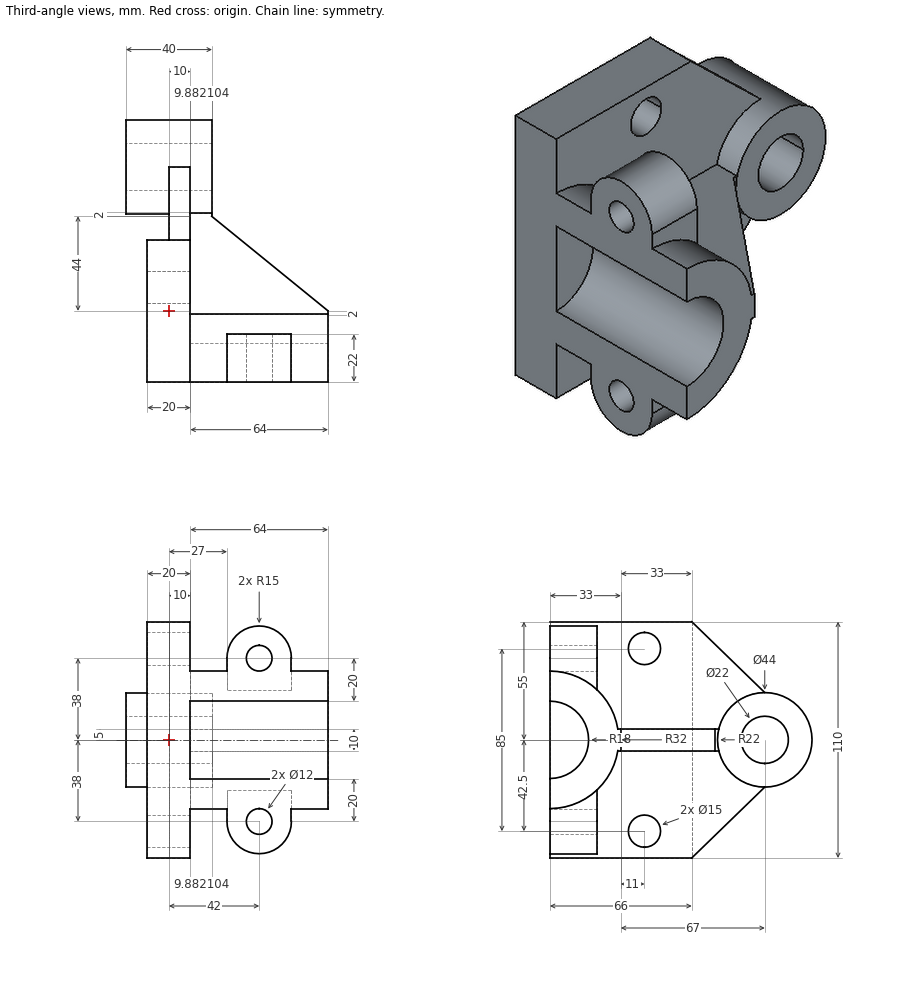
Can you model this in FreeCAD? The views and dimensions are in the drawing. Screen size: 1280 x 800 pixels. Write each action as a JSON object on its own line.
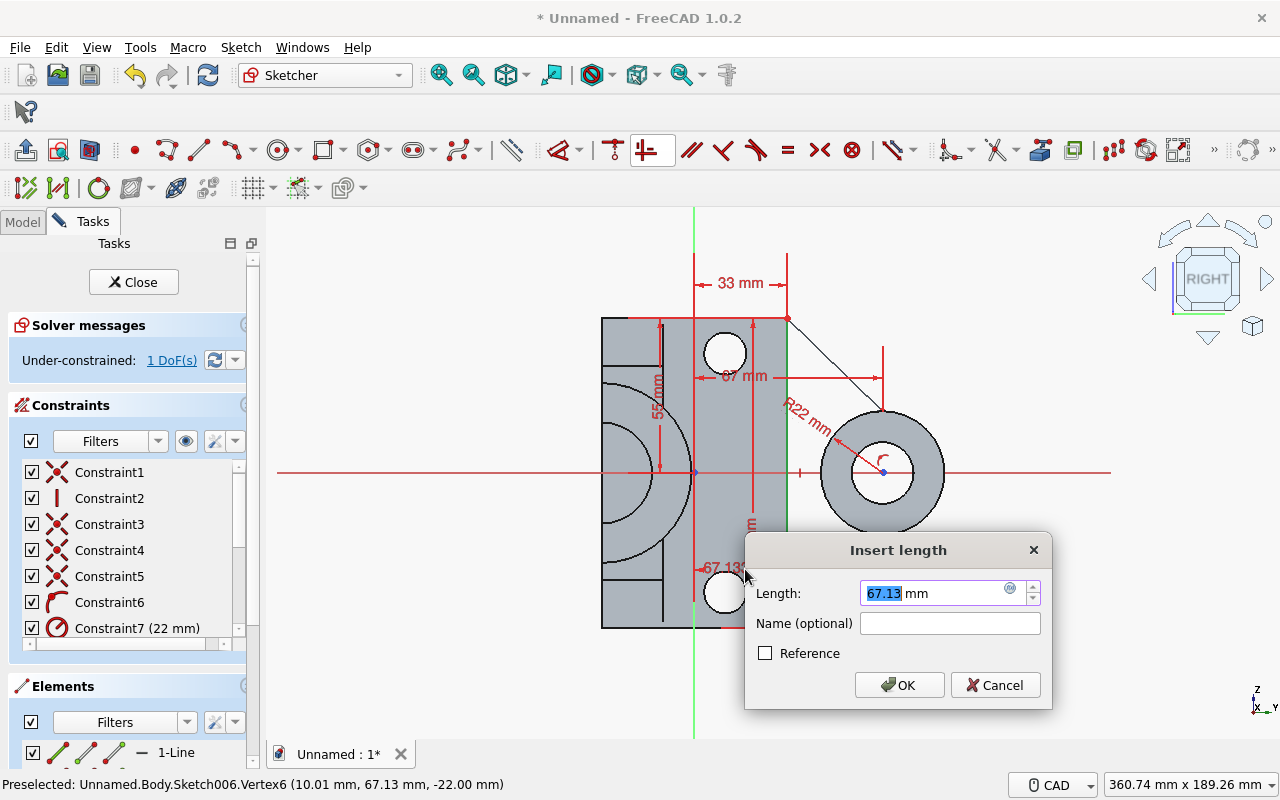
{"action": "type", "text": "67"}
{"action": "key", "text": "Return"}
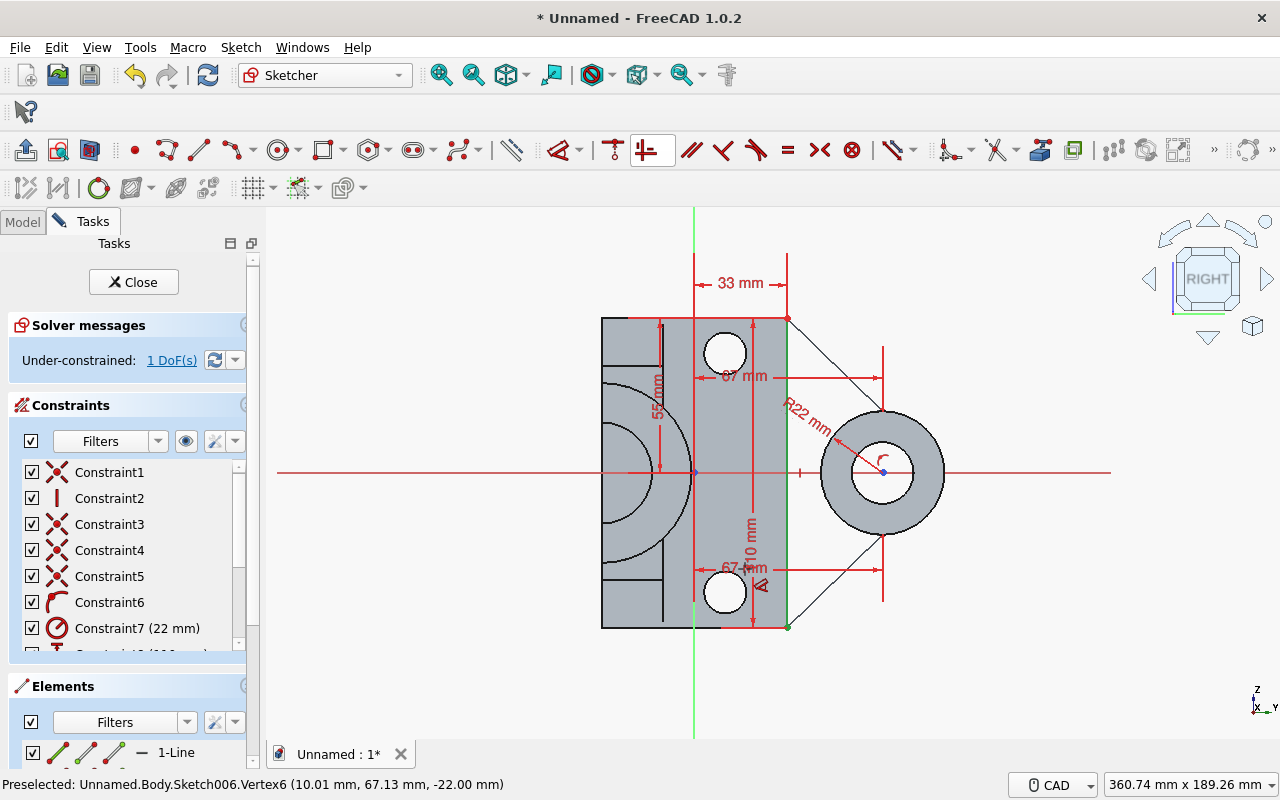
{"action": "left_click", "coordinate": [883, 473]}
{"action": "left_click", "coordinate": [745, 507]}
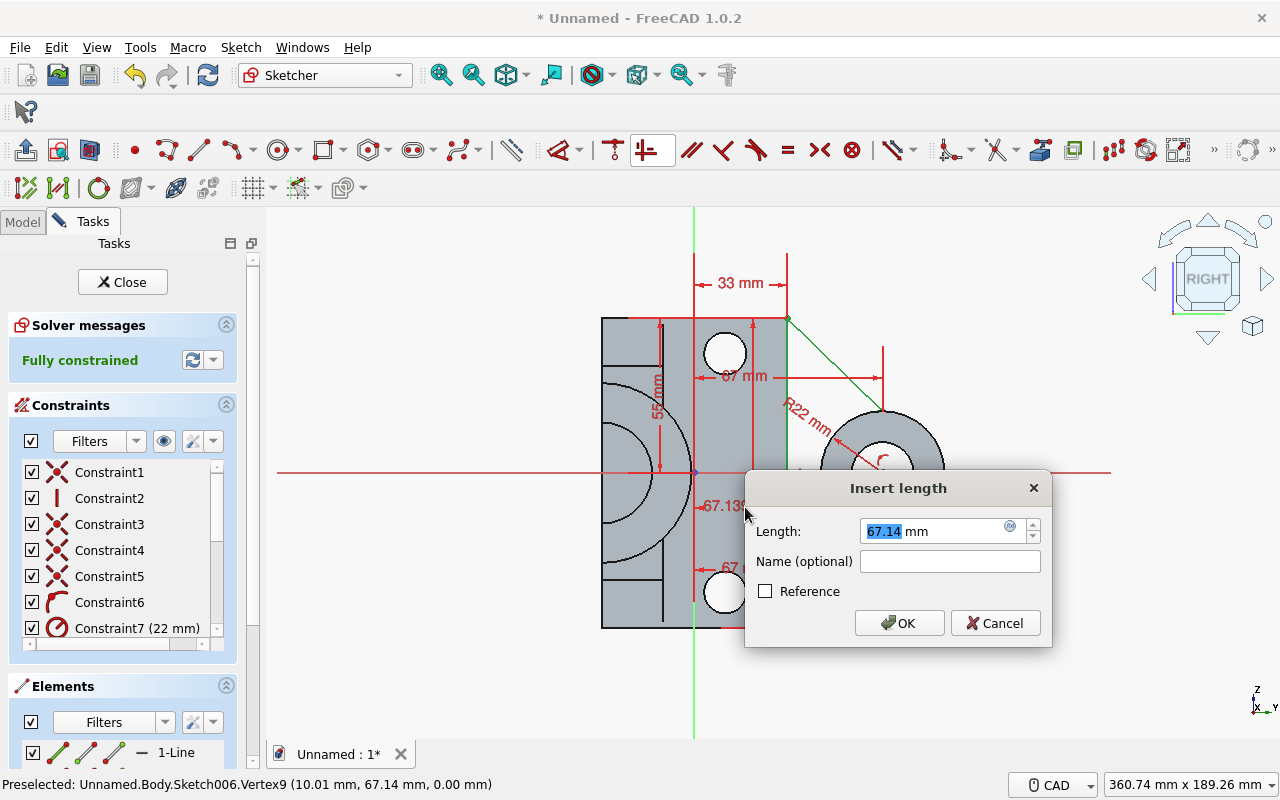
{"action": "type", "text": "67"}
{"action": "key", "text": "Return"}
{"action": "key", "text": "Escape"}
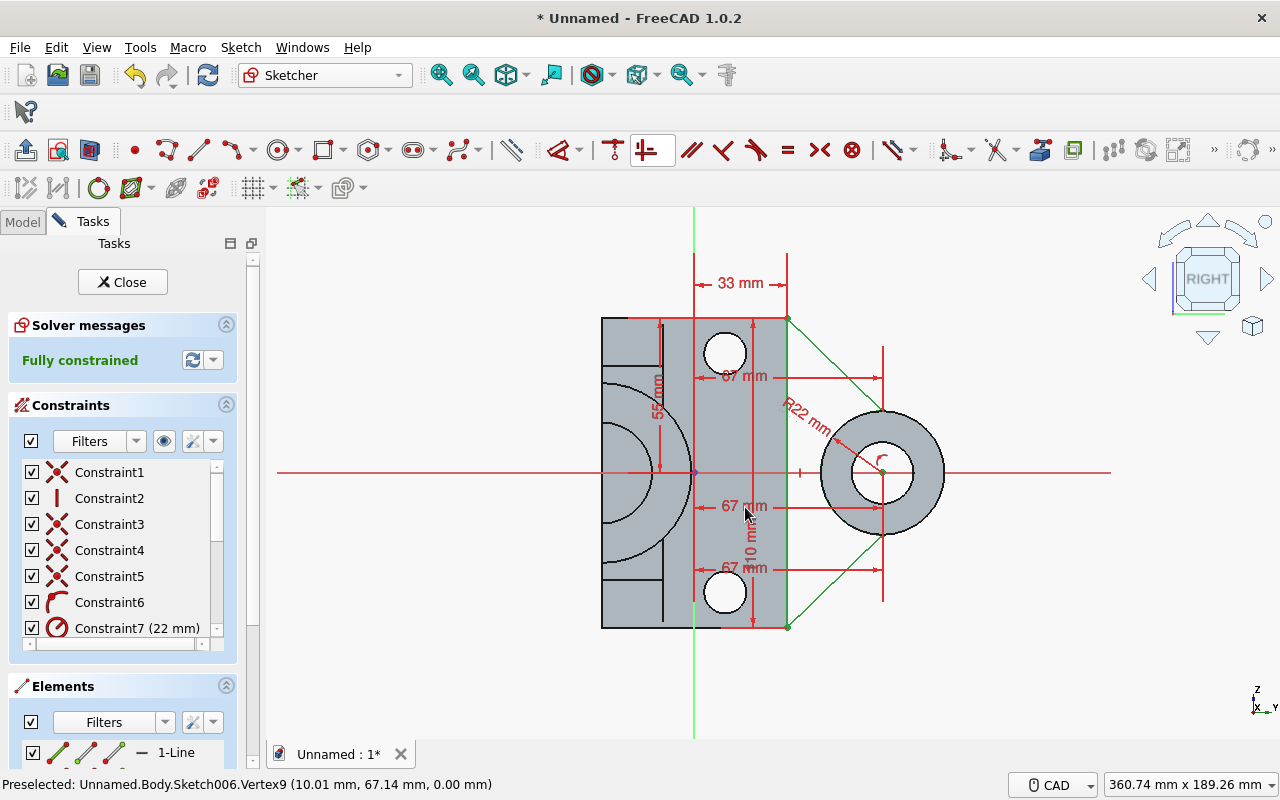
{"action": "left_click", "coordinate": [123, 282]}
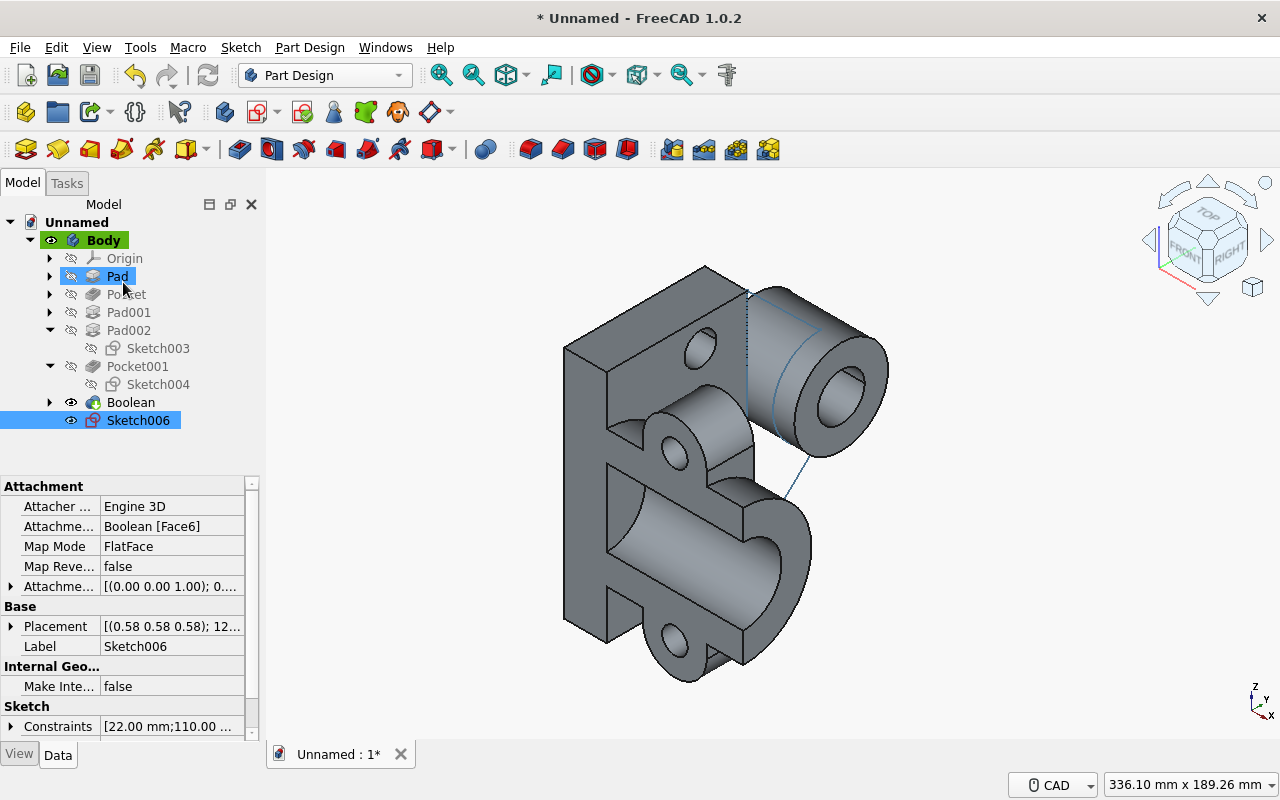
{"action": "left_click", "coordinate": [26, 150]}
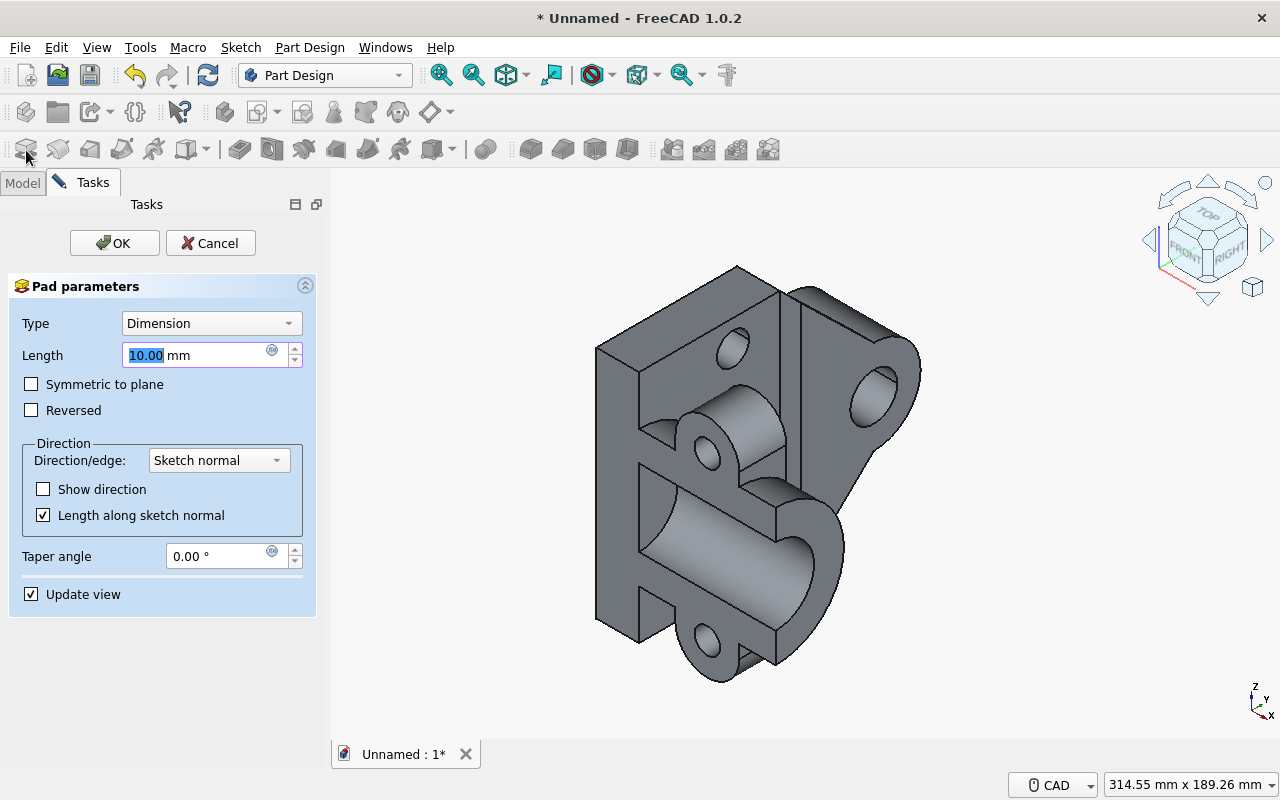
{"action": "type", "text": "10"}
{"action": "key", "text": "Tab"}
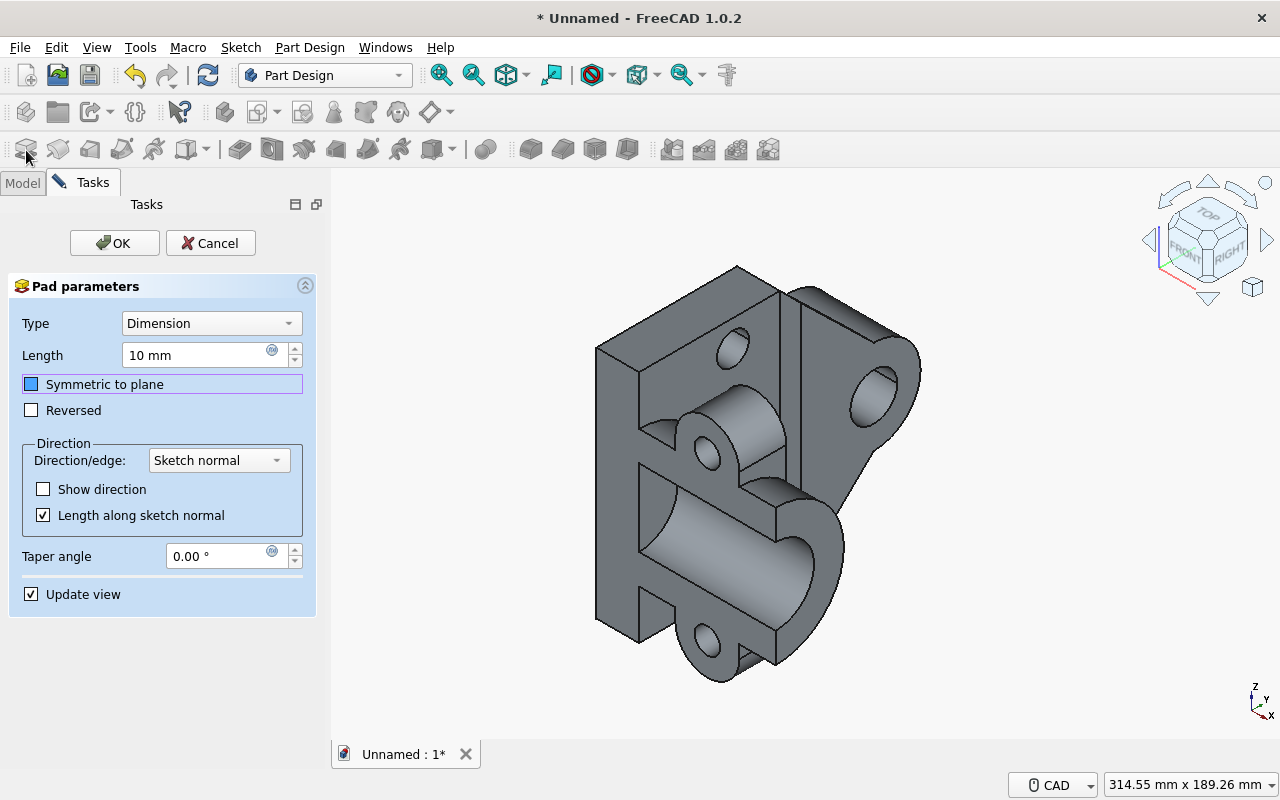
{"action": "left_click", "coordinate": [30, 410]}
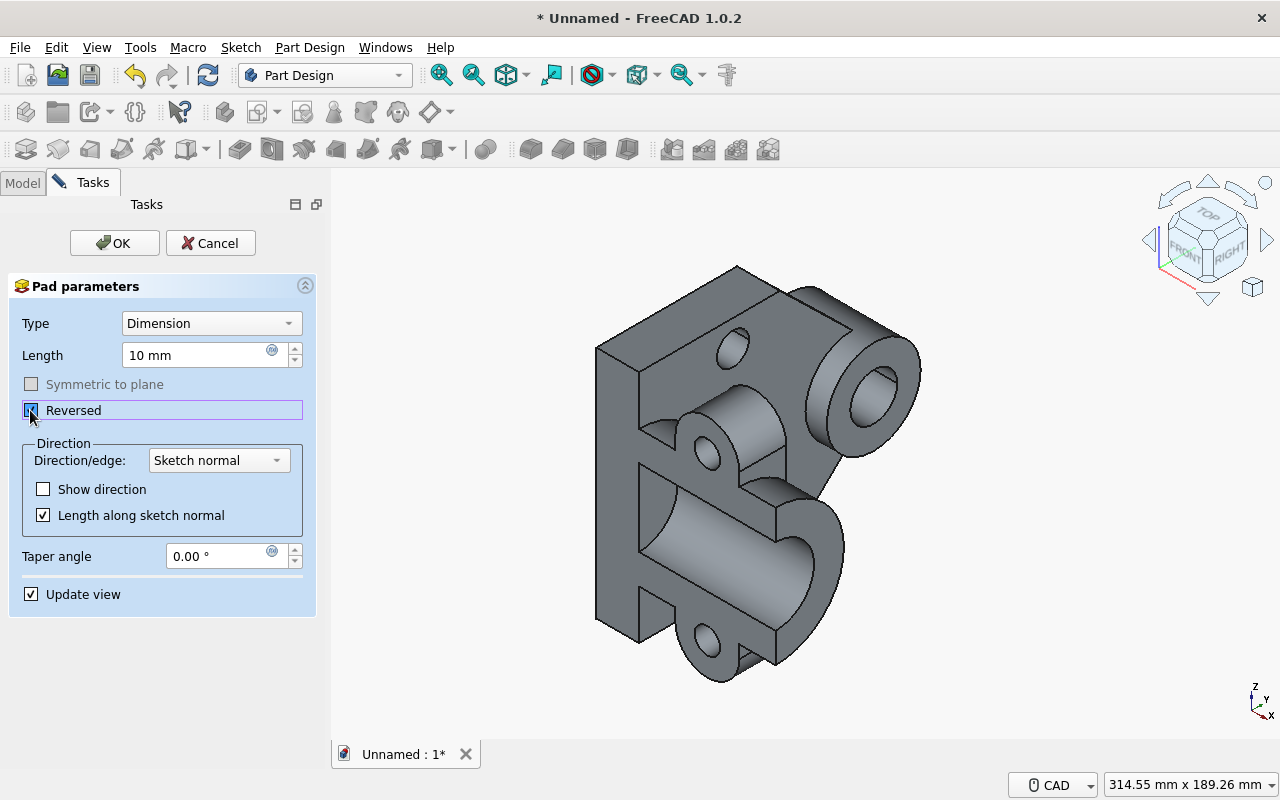
{"action": "left_click", "coordinate": [115, 243]}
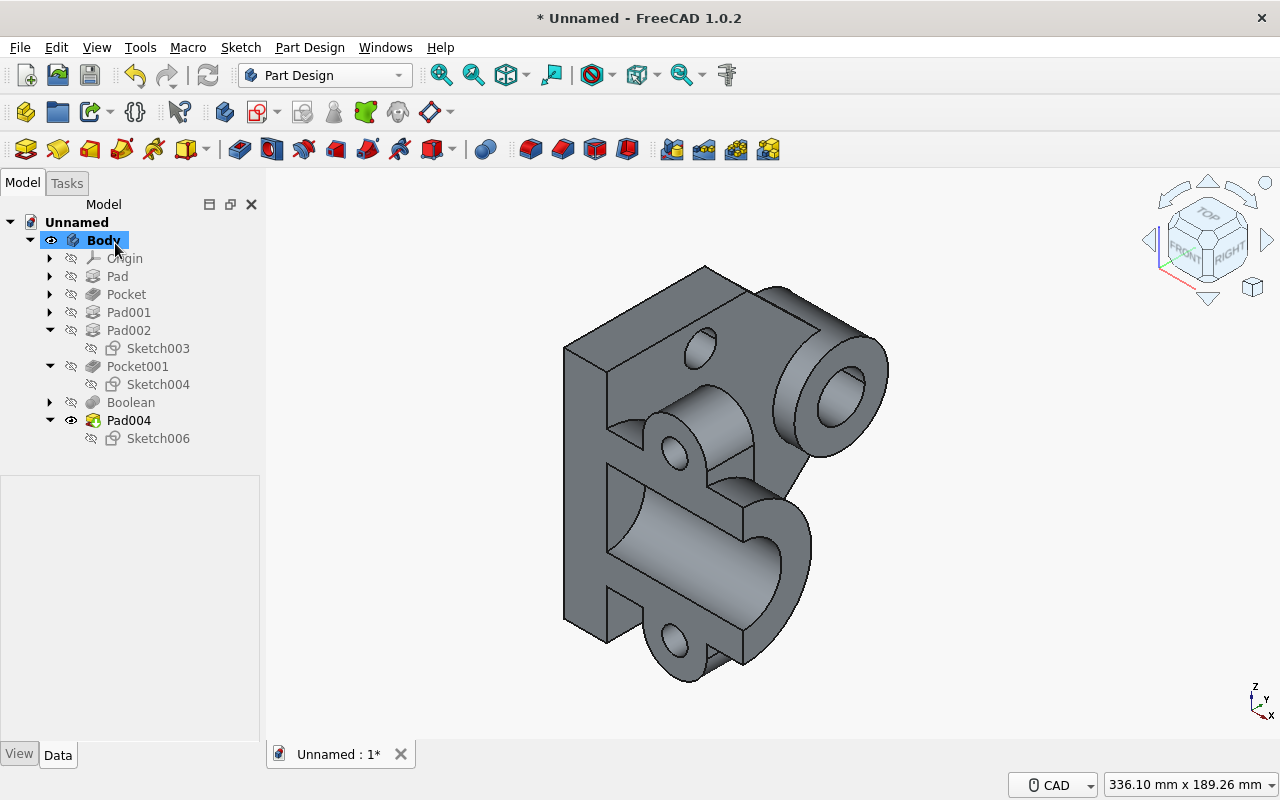
{"action": "left_click", "coordinate": [258, 112]}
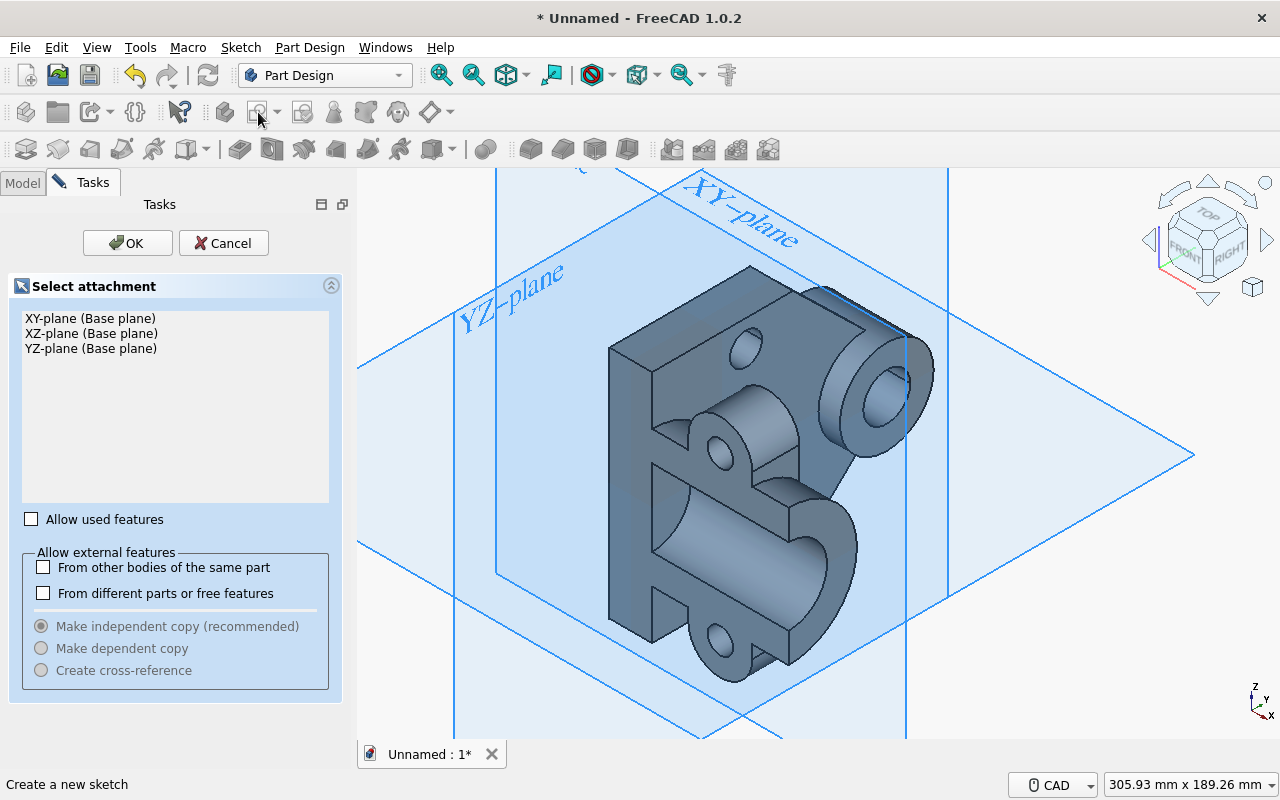
{"action": "left_click", "coordinate": [82, 318]}